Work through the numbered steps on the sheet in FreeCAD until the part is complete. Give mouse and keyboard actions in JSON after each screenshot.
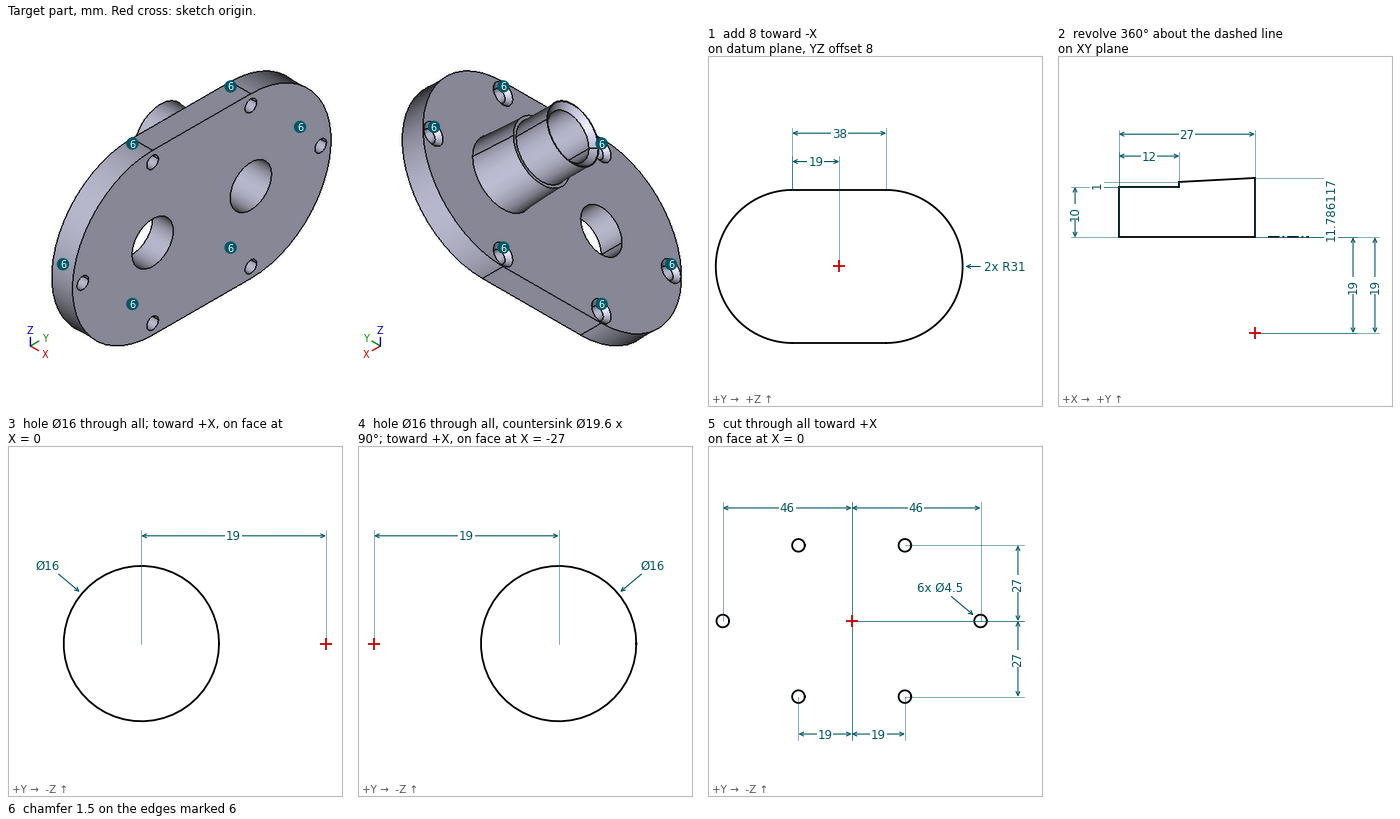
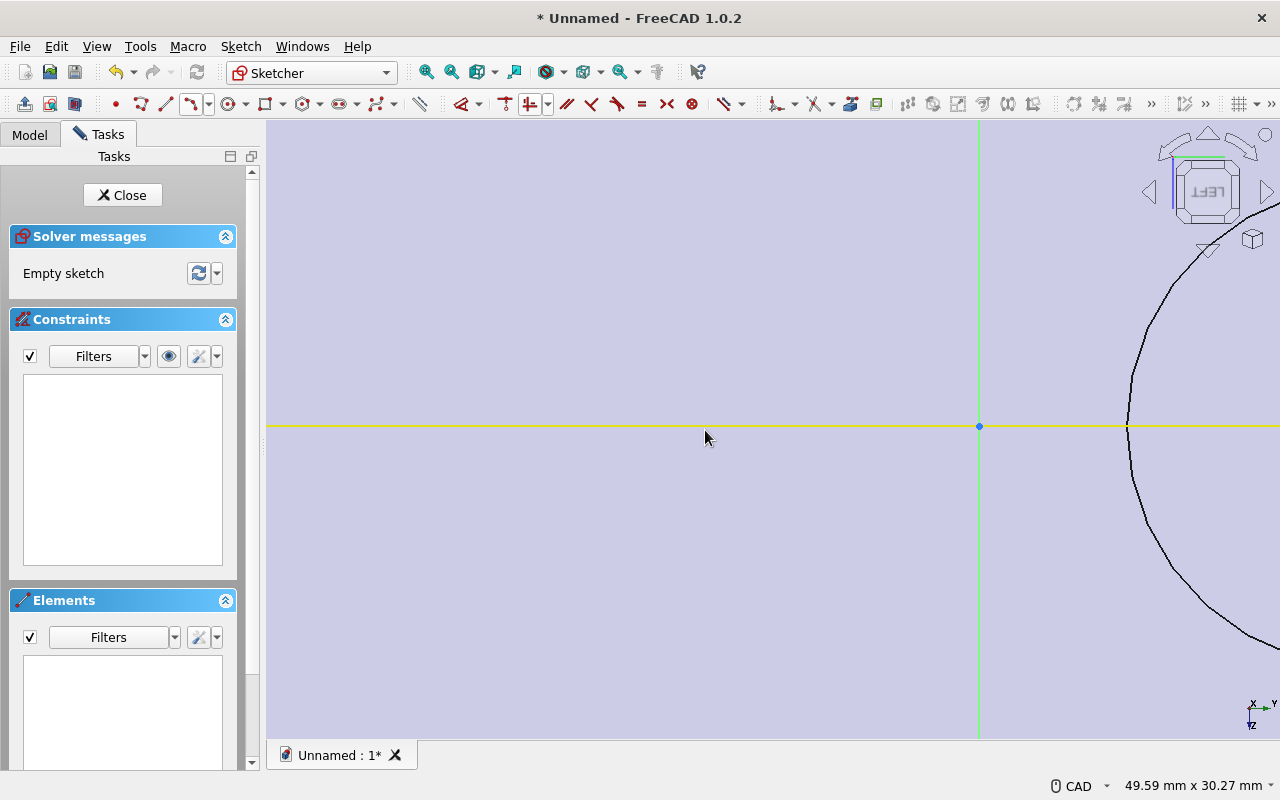
{"action": "left_click", "coordinate": [228, 104]}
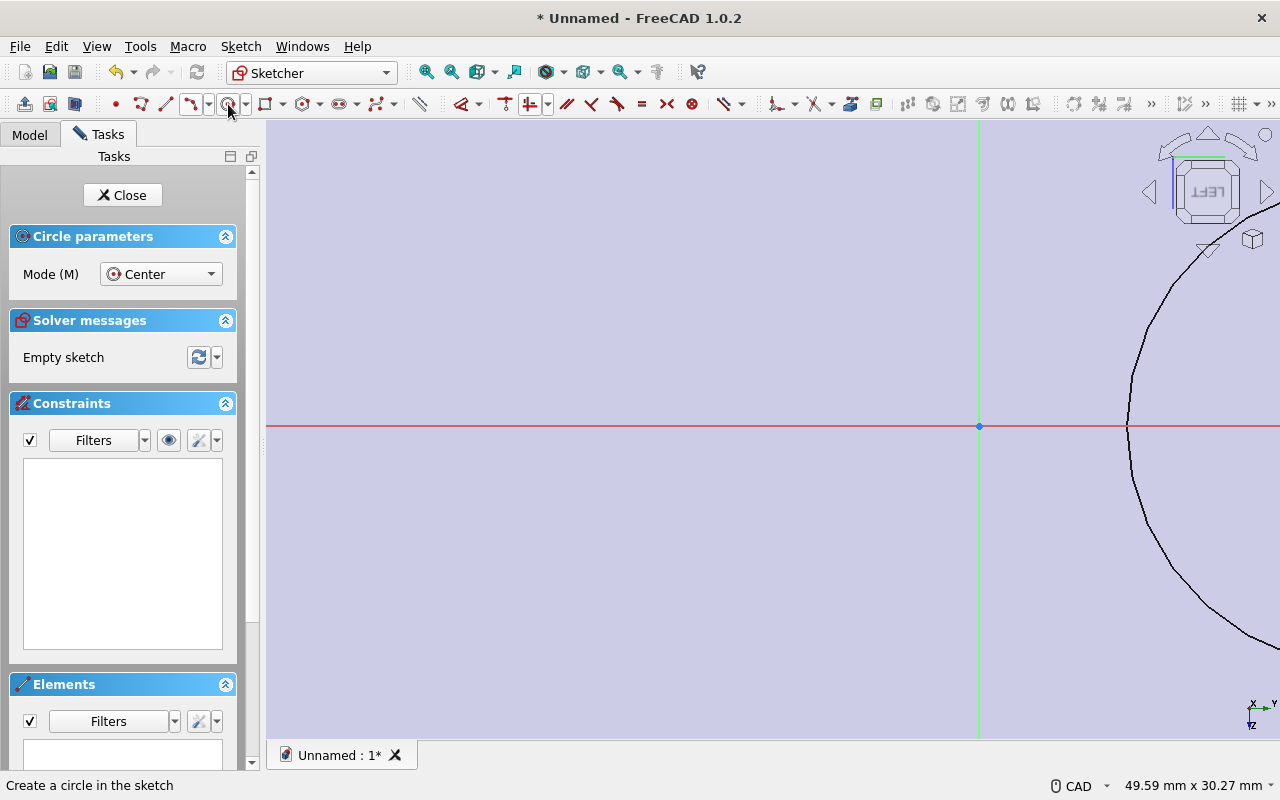
{"action": "left_click", "coordinate": [591, 426]}
{"action": "left_click", "coordinate": [707, 311]}
{"action": "key", "text": "Escape"}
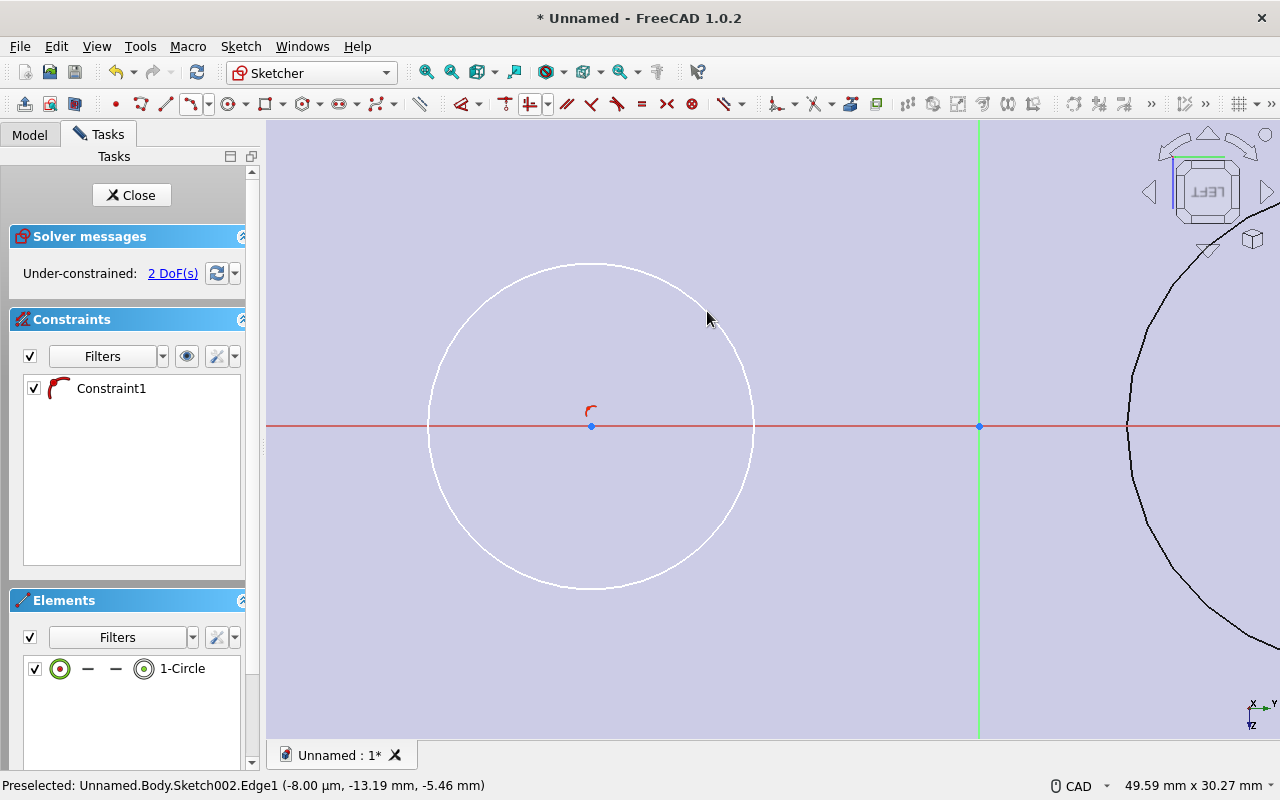
{"action": "key", "text": "d"}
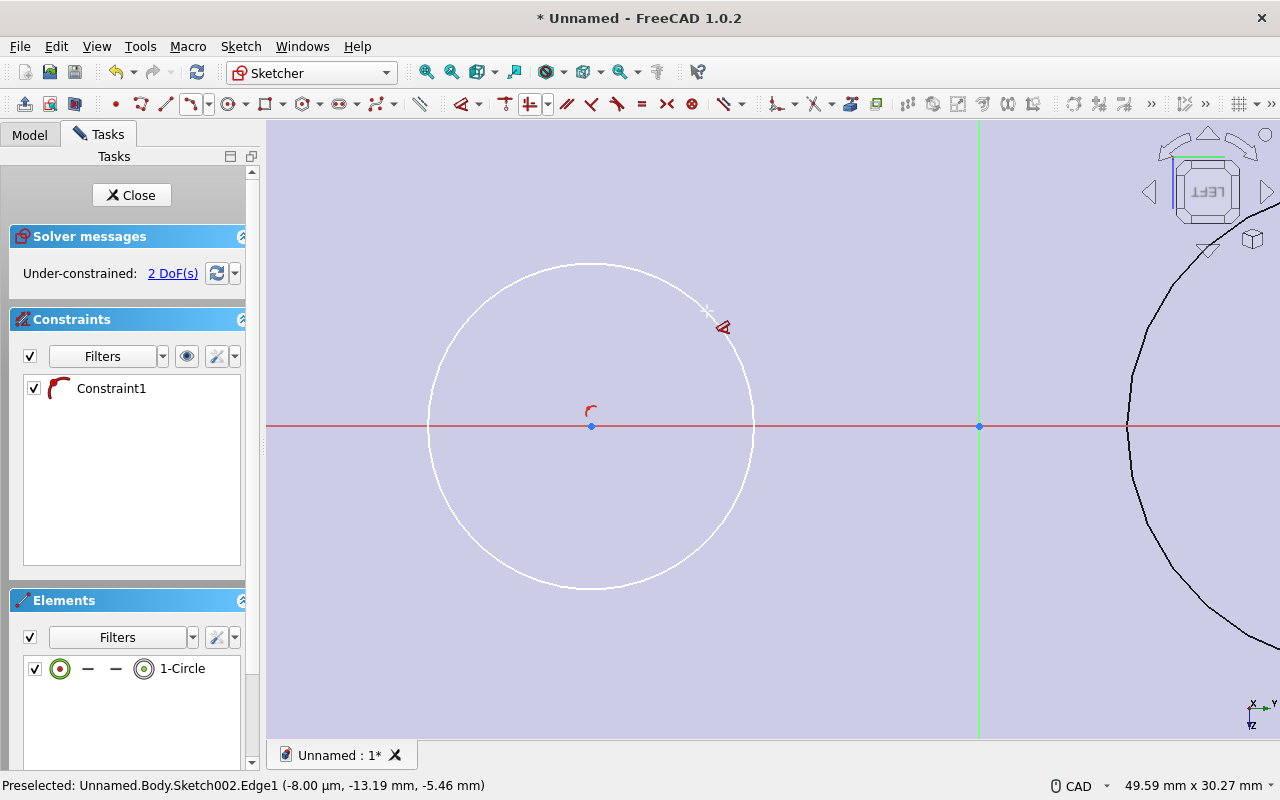
{"action": "left_click", "coordinate": [706, 311]}
{"action": "left_click", "coordinate": [729, 288]}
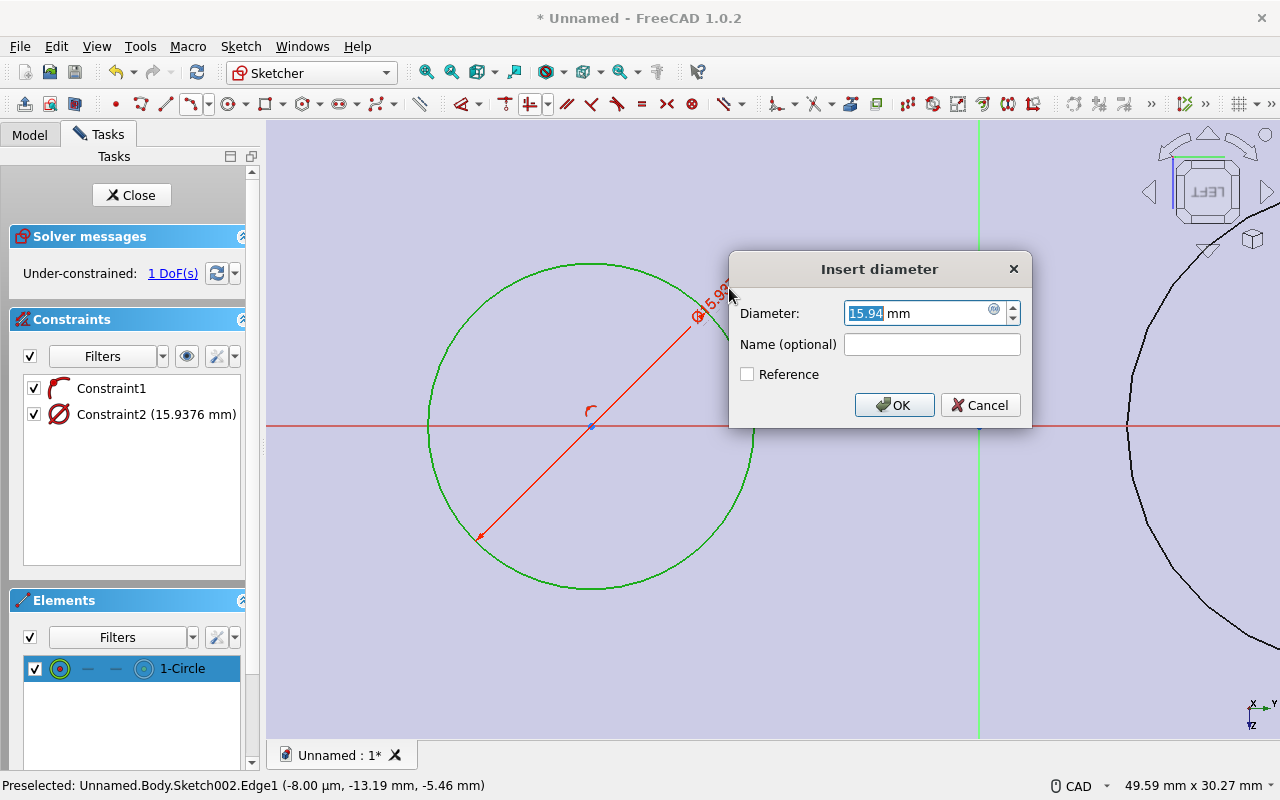
{"action": "type", "text": "16"}
{"action": "key", "text": "Return"}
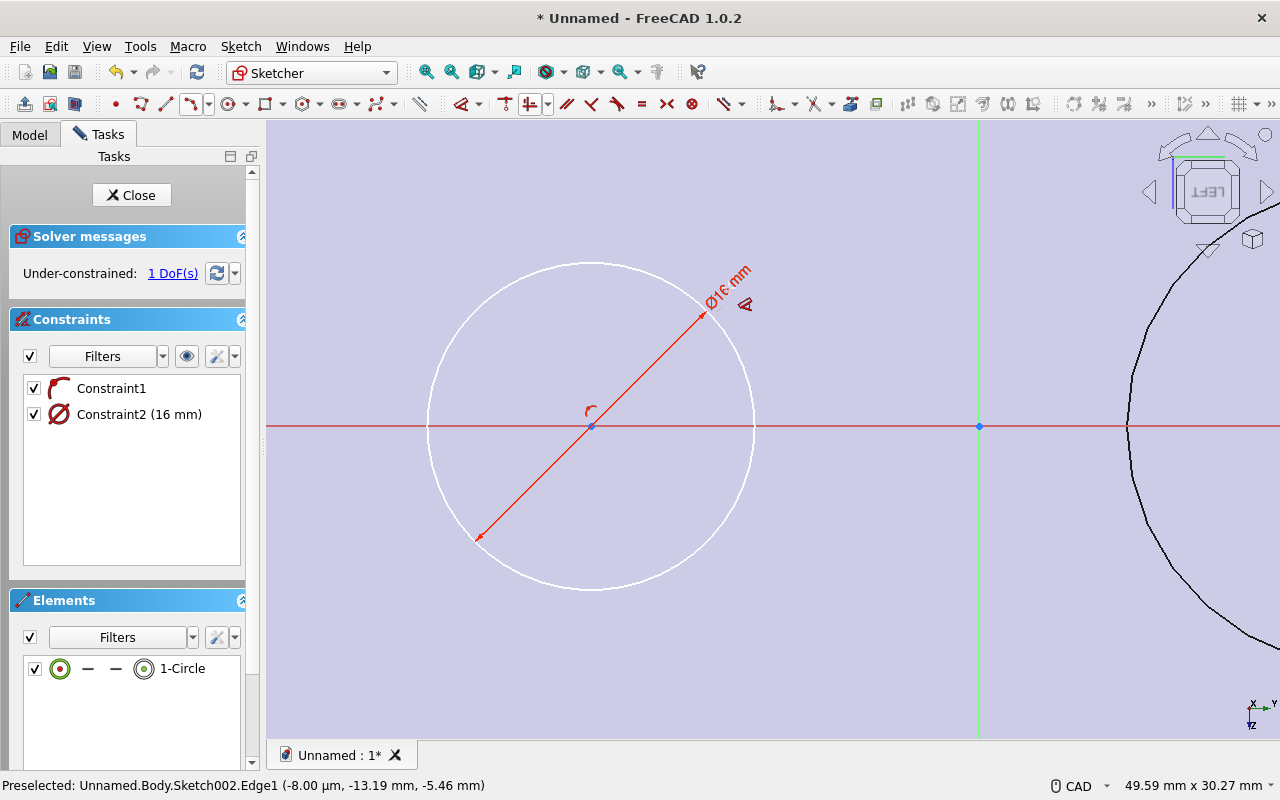
{"action": "left_click", "coordinate": [591, 426]}
{"action": "left_click", "coordinate": [785, 460]}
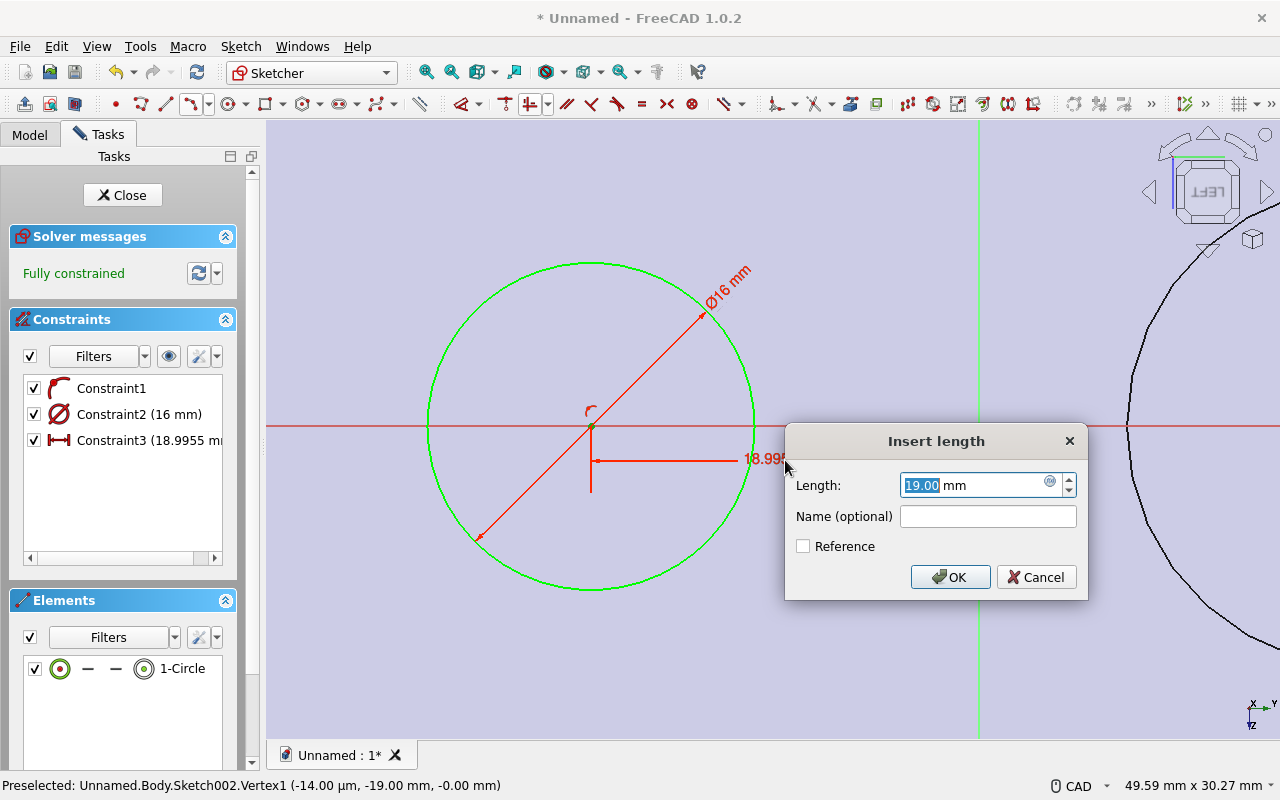
{"action": "type", "text": "19"}
{"action": "key", "text": "Return"}
{"action": "key", "text": "Escape"}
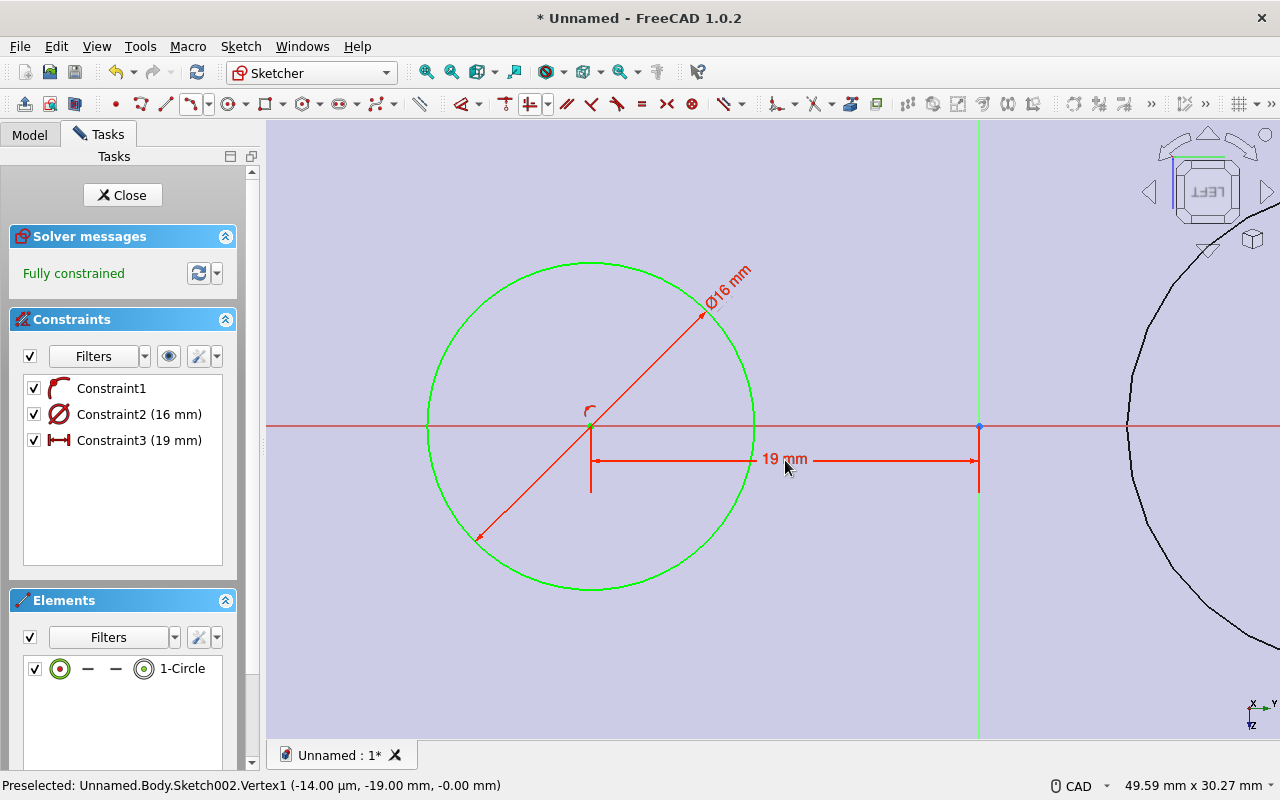
{"action": "left_click", "coordinate": [123, 195]}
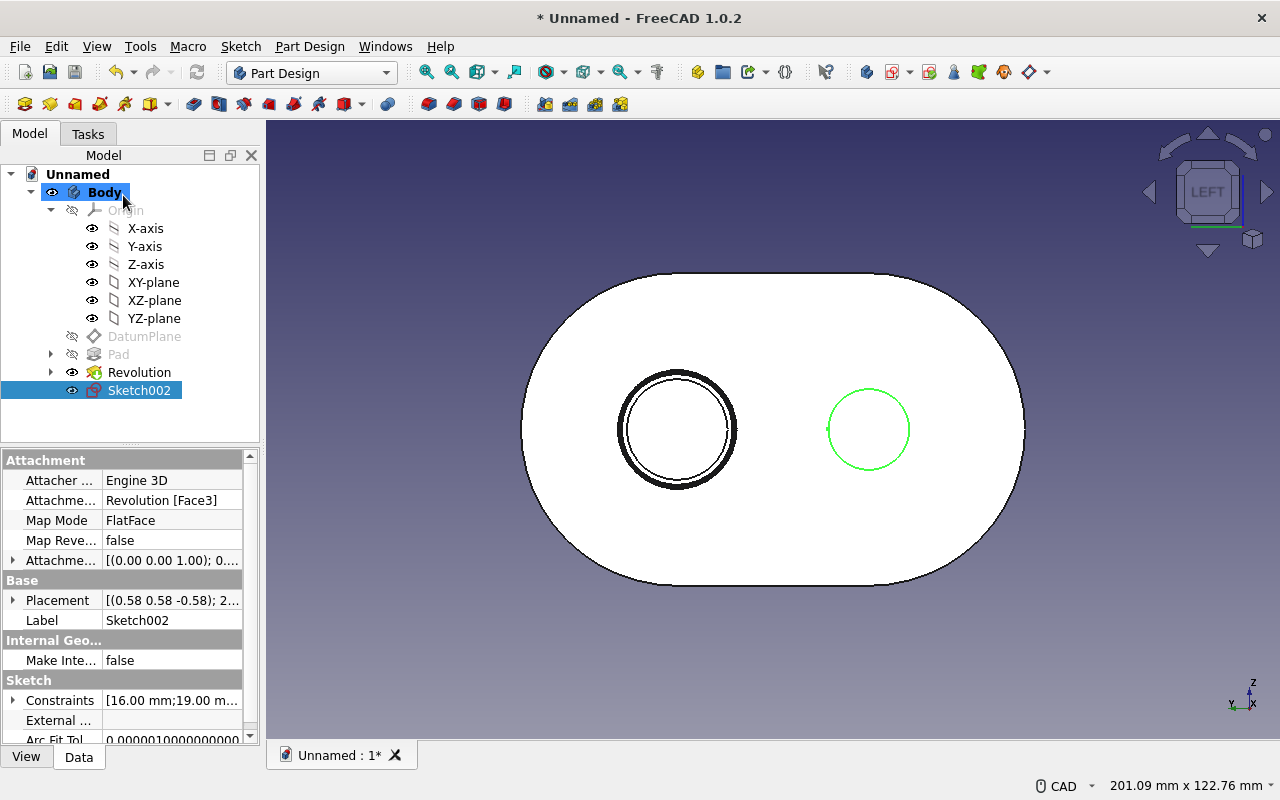
{"action": "left_click", "coordinate": [219, 104]}